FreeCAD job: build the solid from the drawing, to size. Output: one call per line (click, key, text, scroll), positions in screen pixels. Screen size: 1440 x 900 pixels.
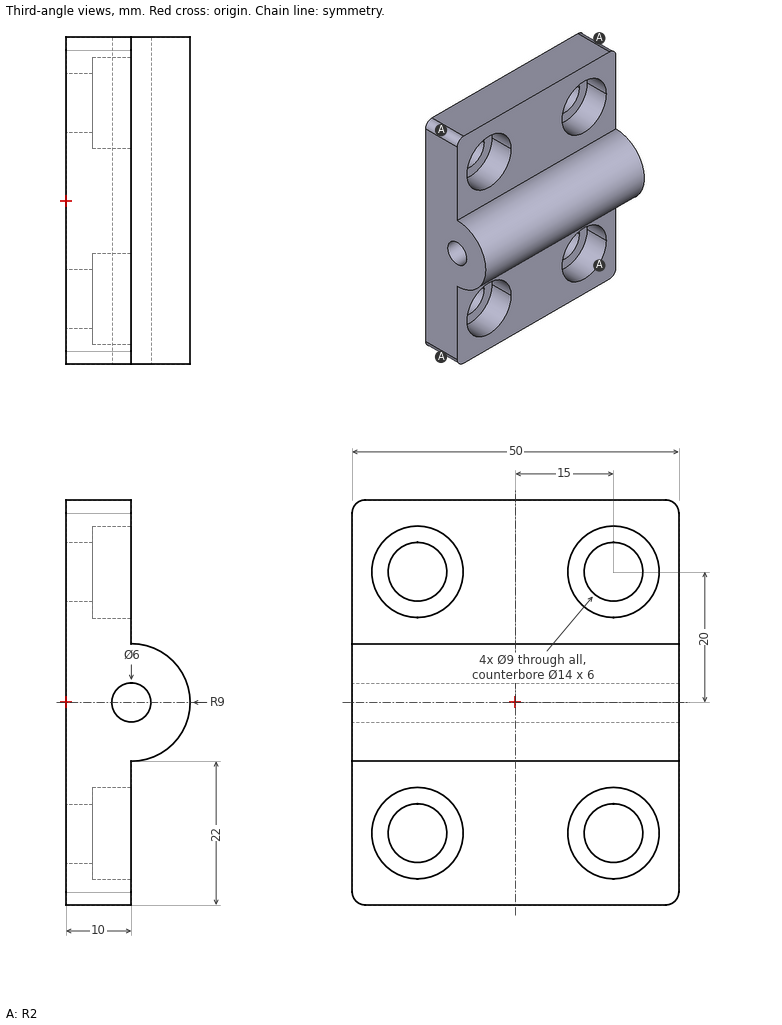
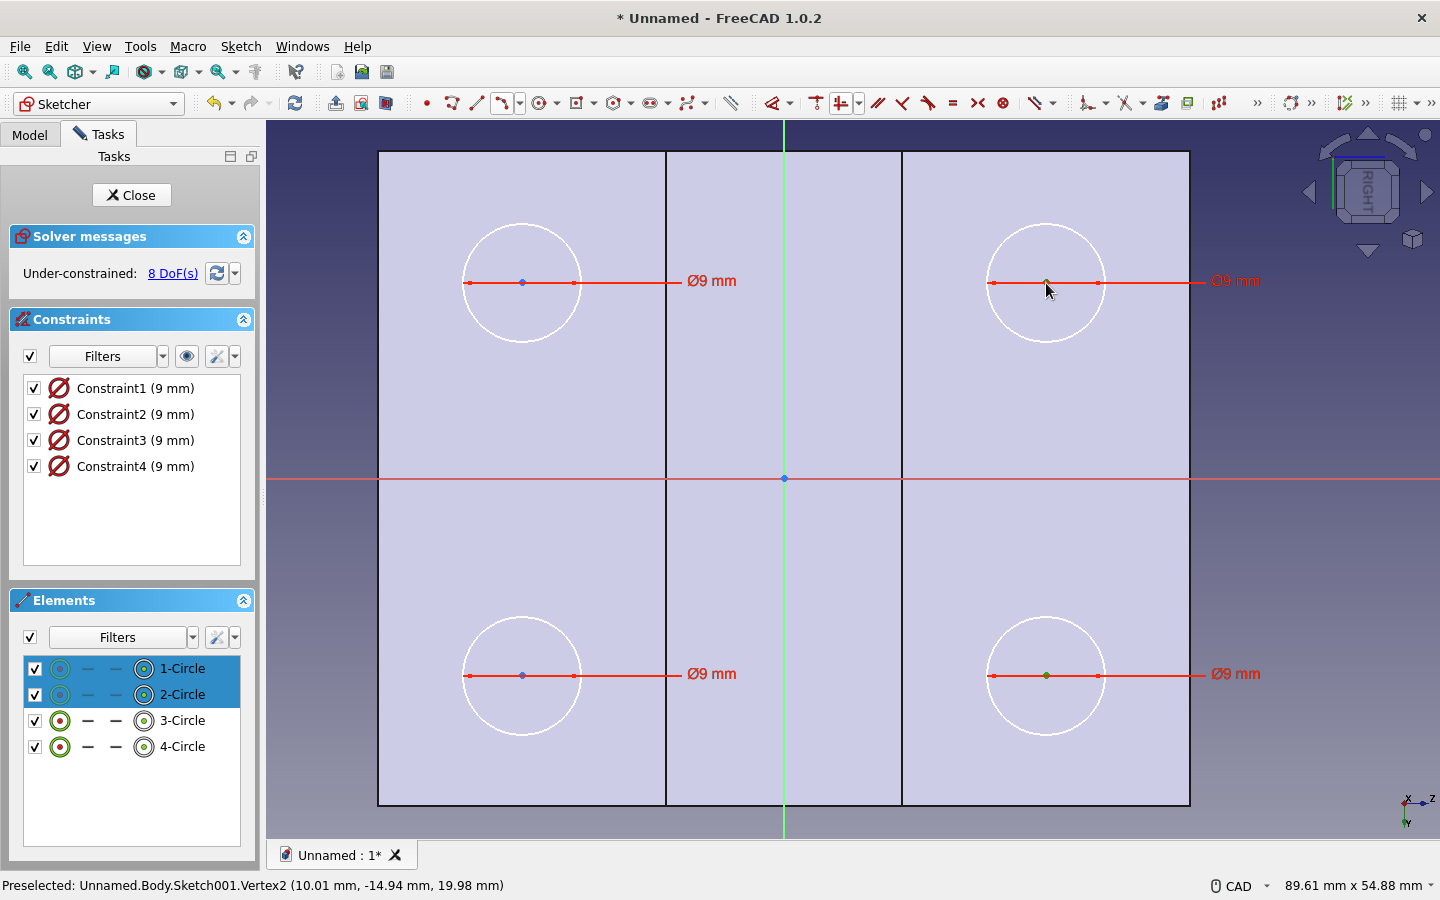
click(364, 479)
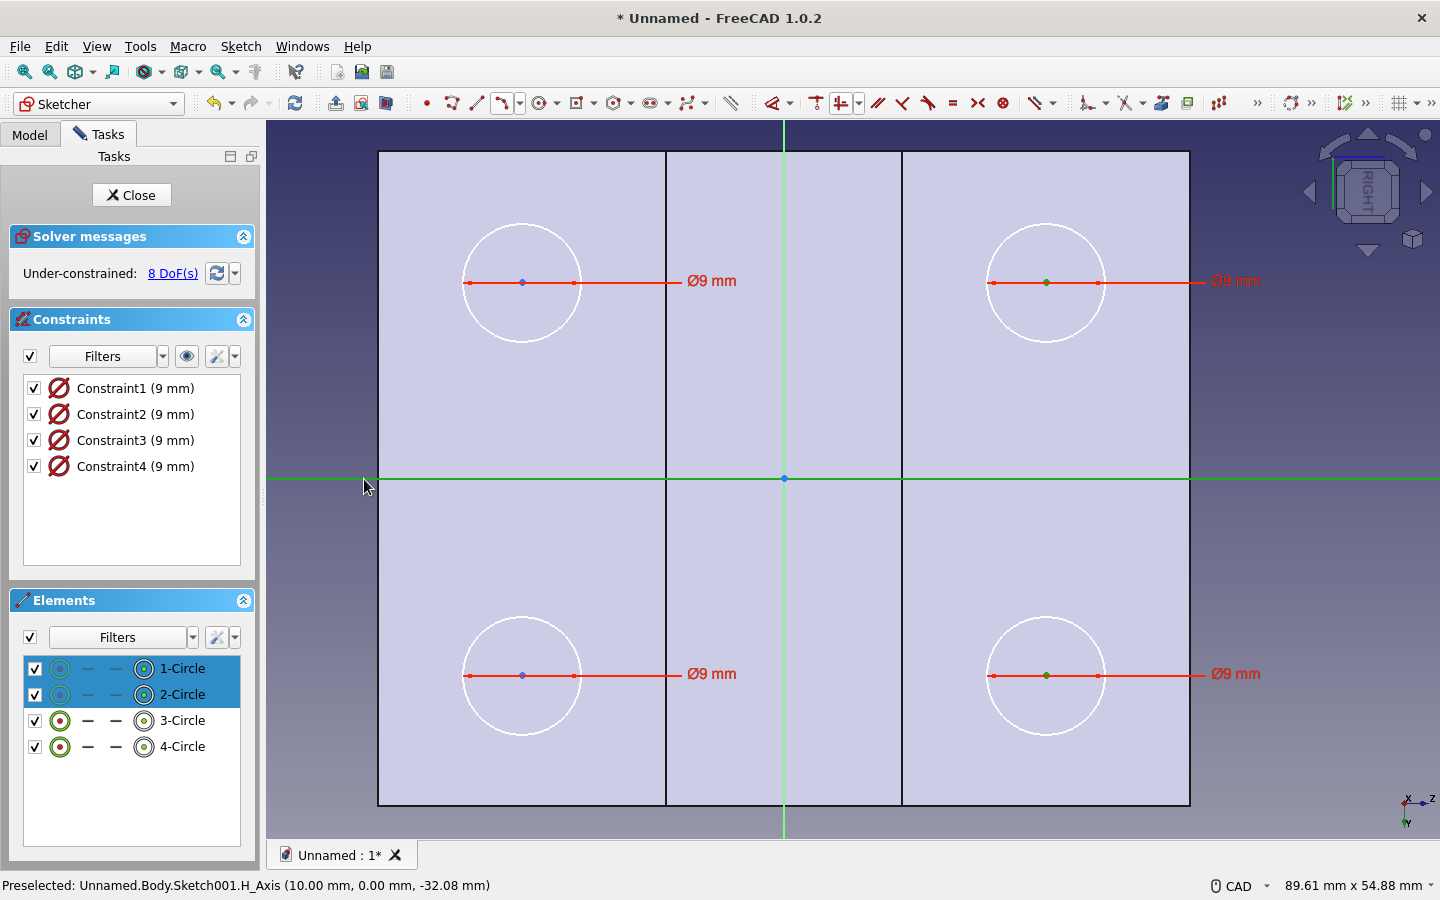
click(978, 104)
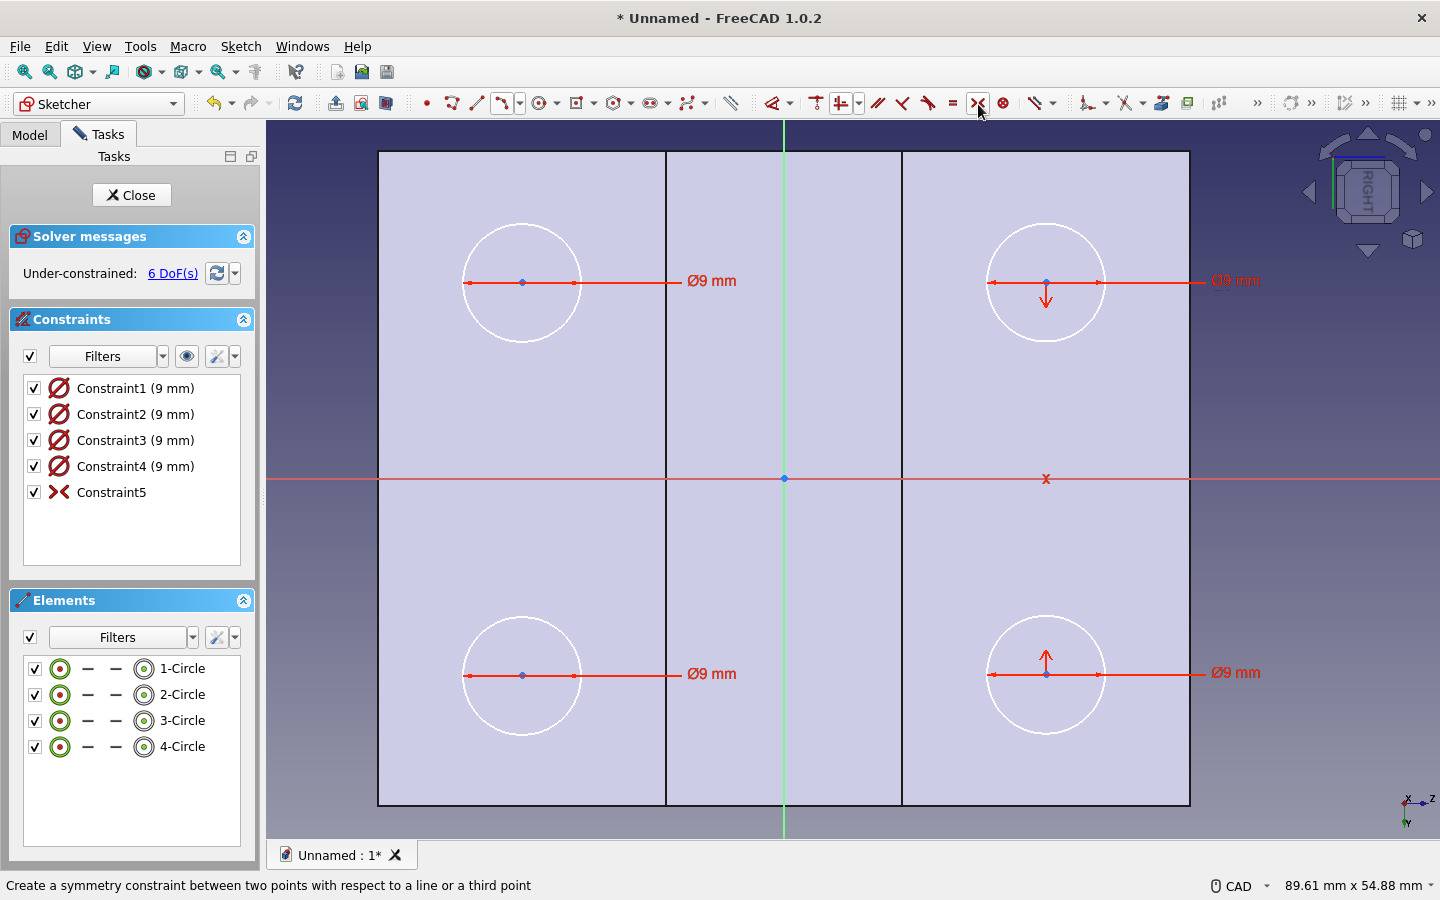
click(1046, 283)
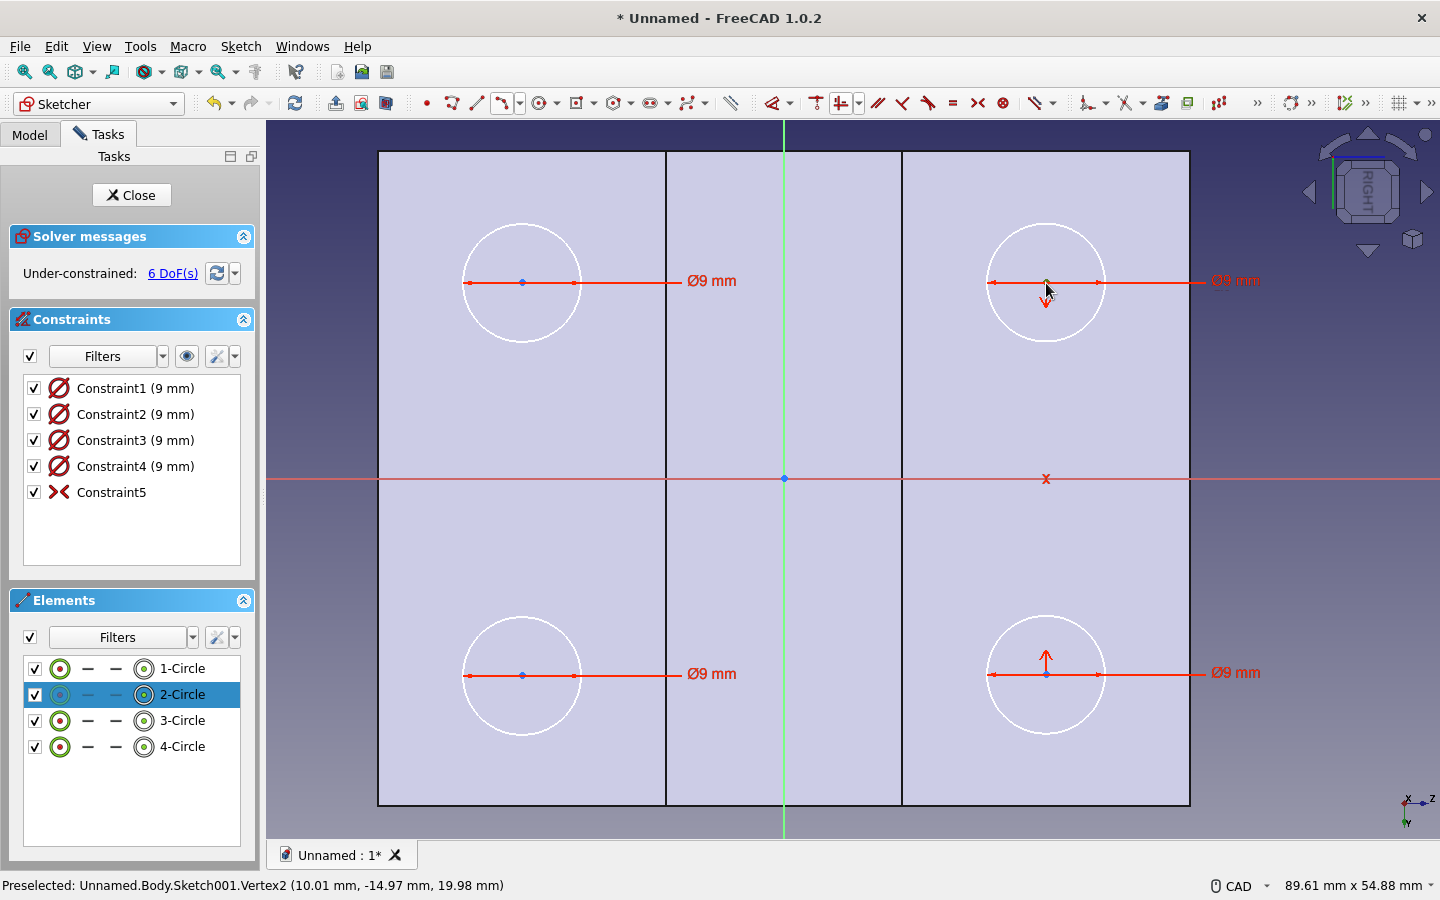
click(522, 283)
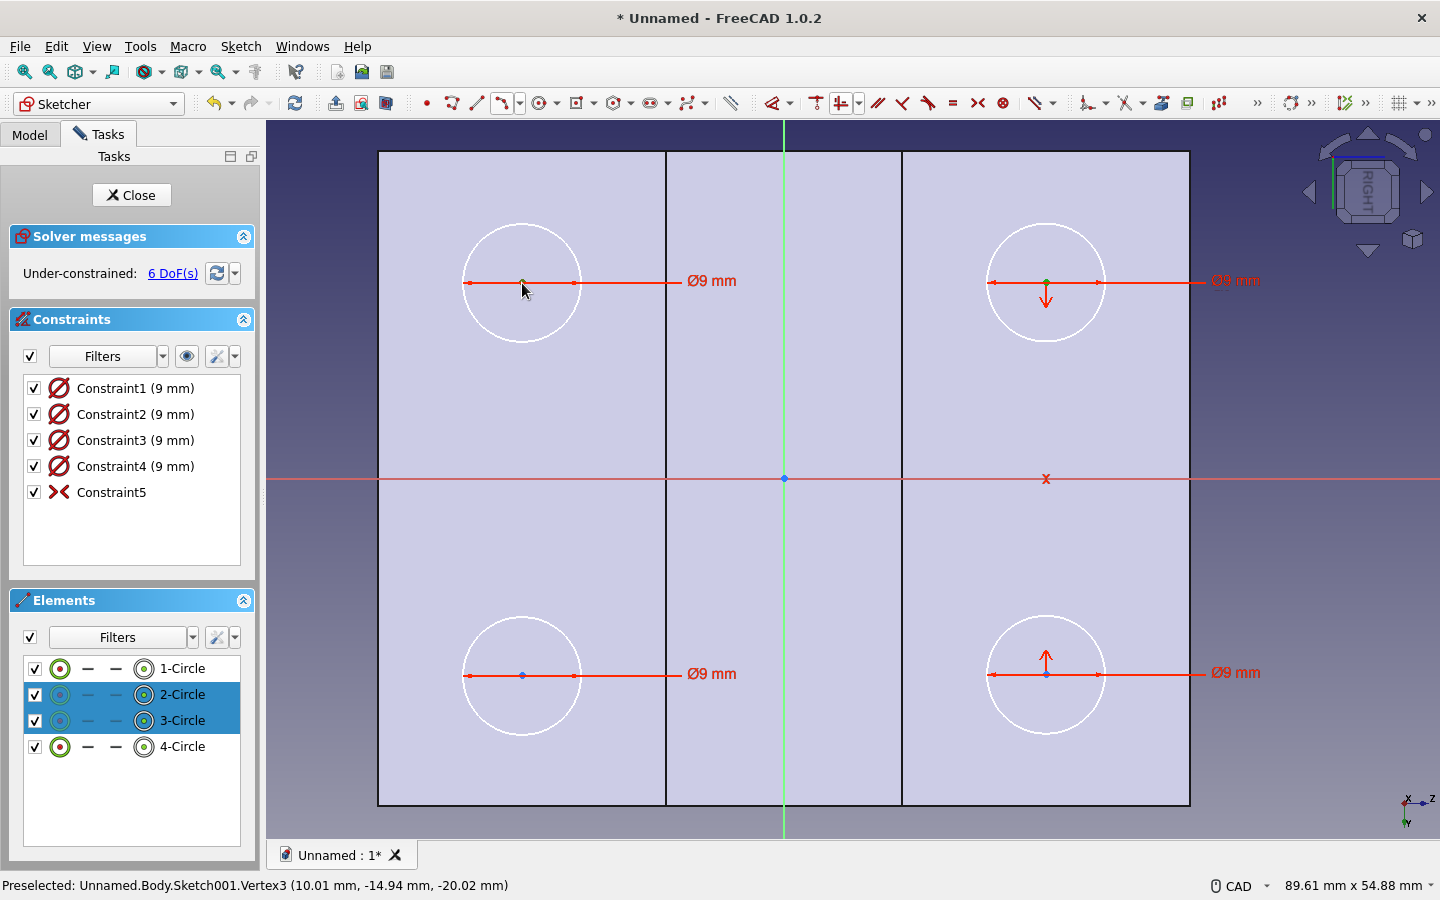
click(784, 764)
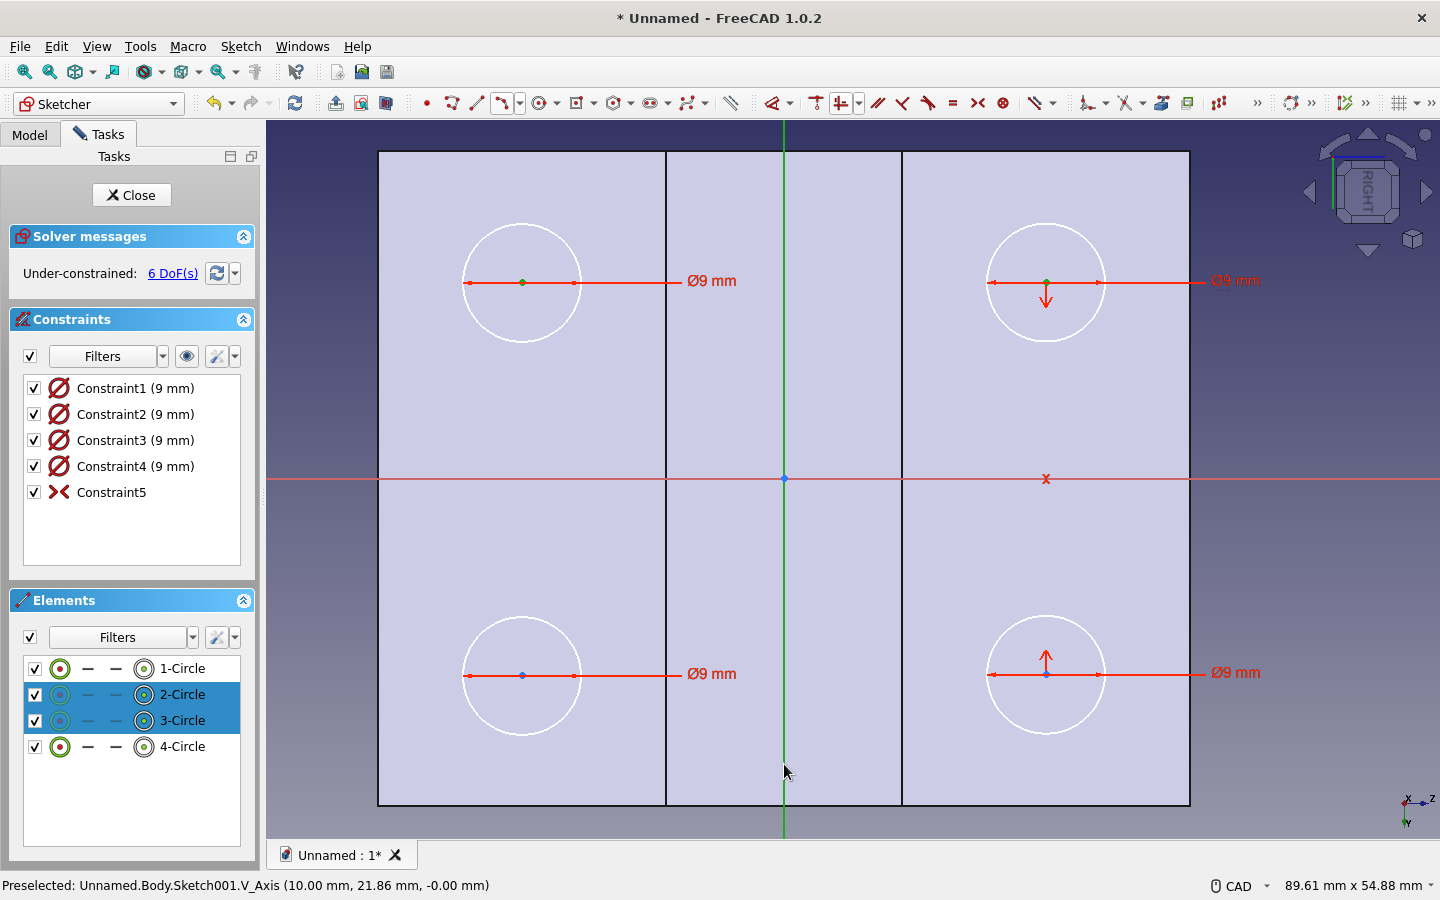
click(978, 104)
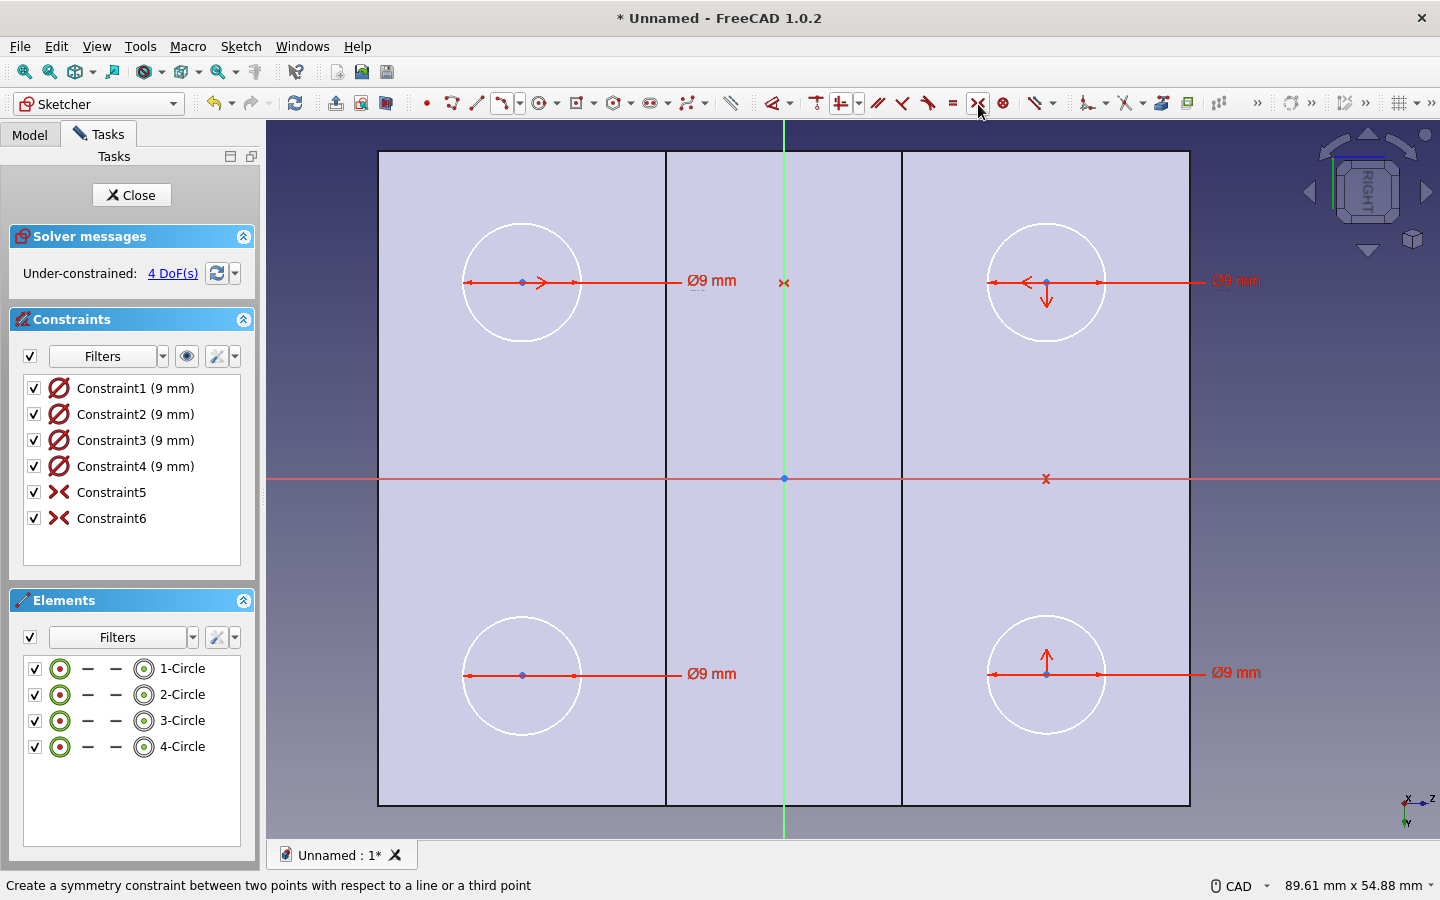
click(1047, 675)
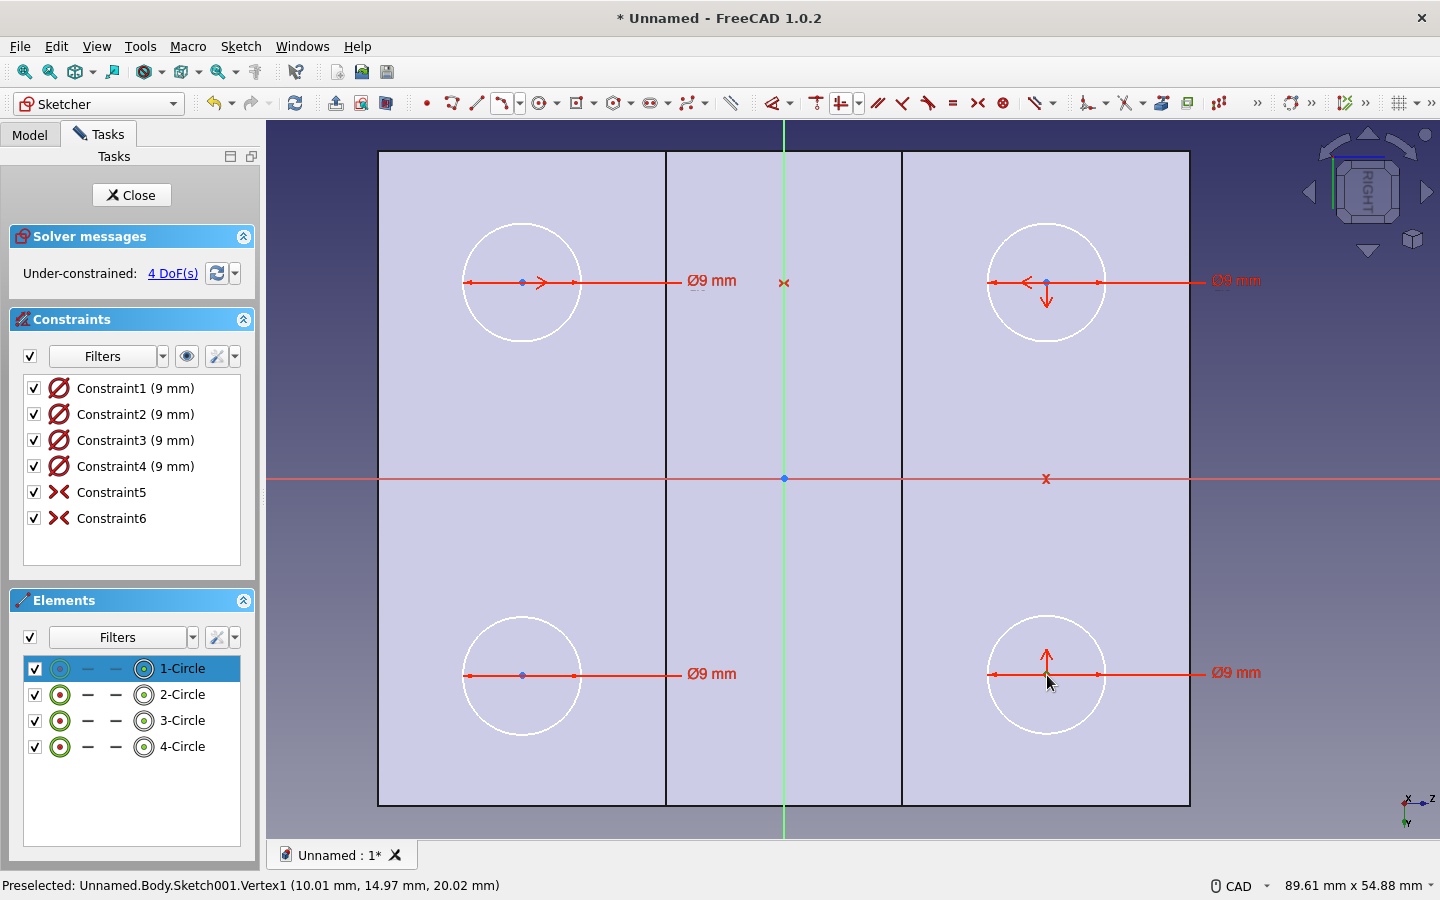
click(522, 676)